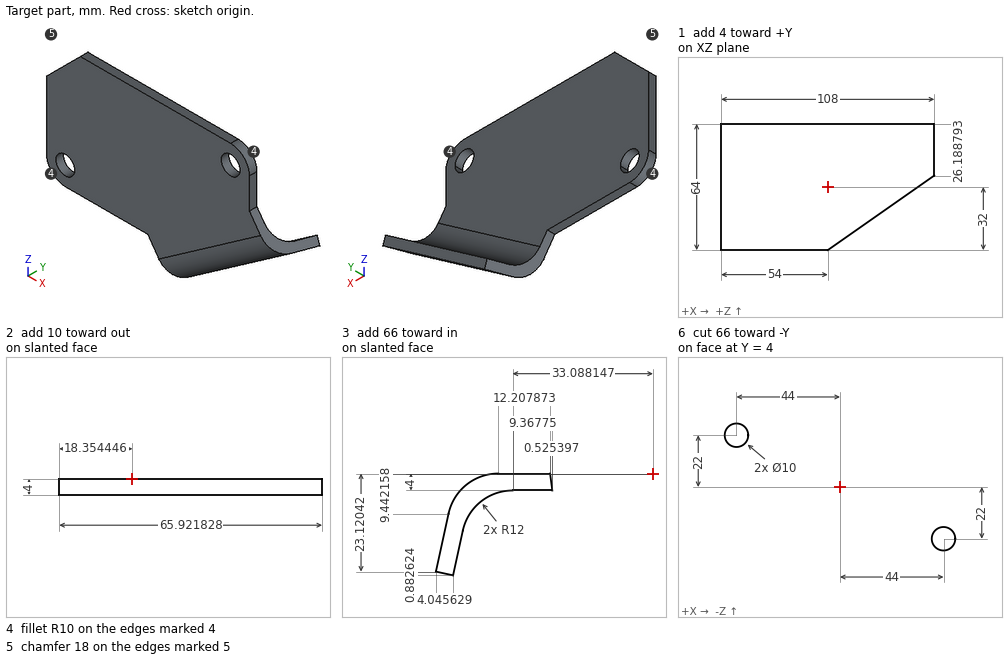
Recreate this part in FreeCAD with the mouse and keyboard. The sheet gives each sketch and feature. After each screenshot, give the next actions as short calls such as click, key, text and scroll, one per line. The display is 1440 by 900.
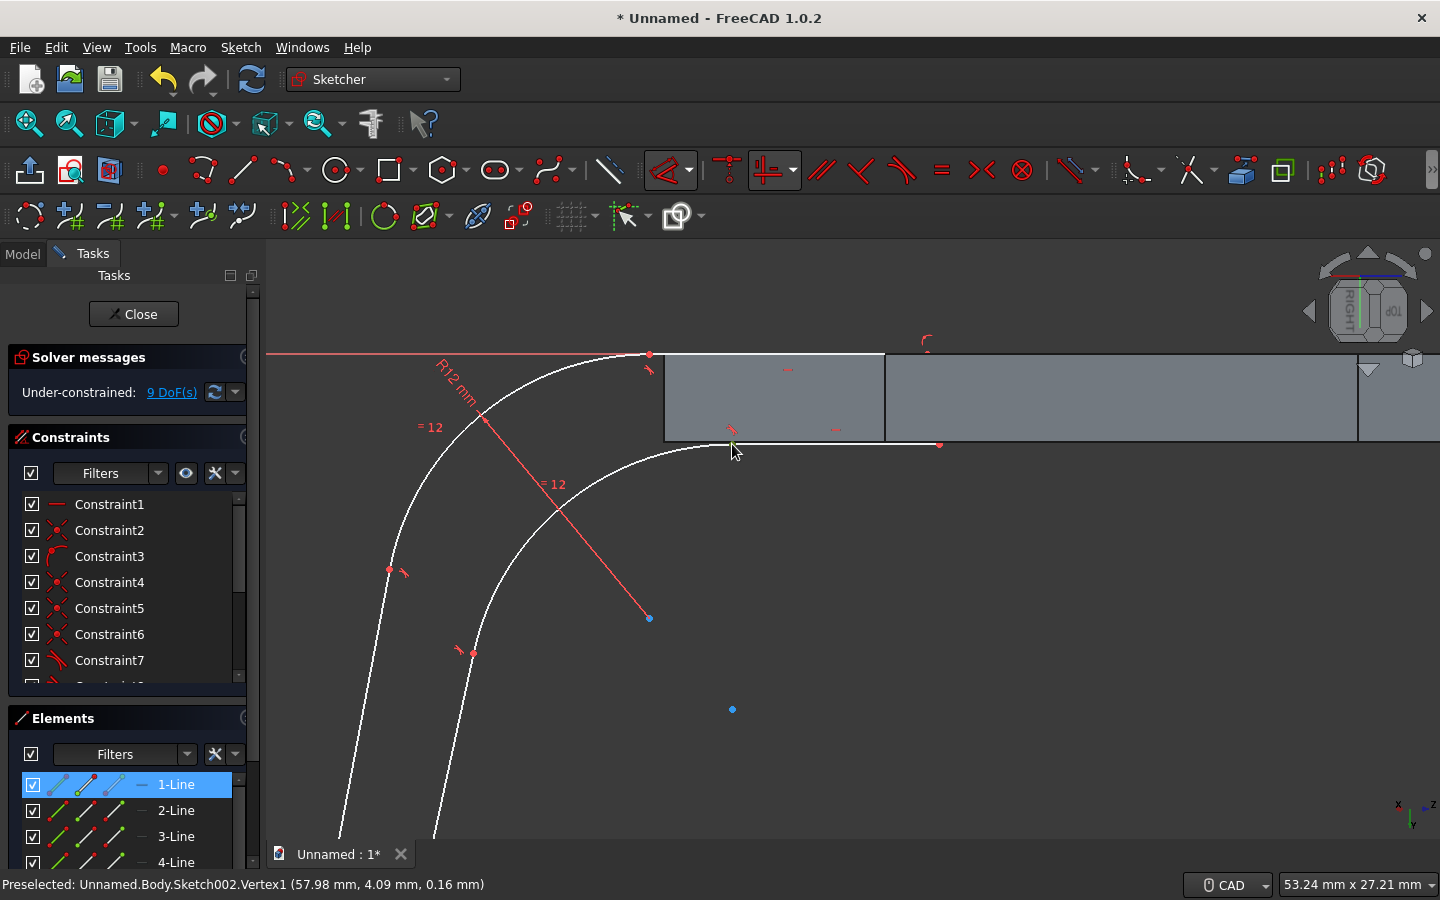
key(i)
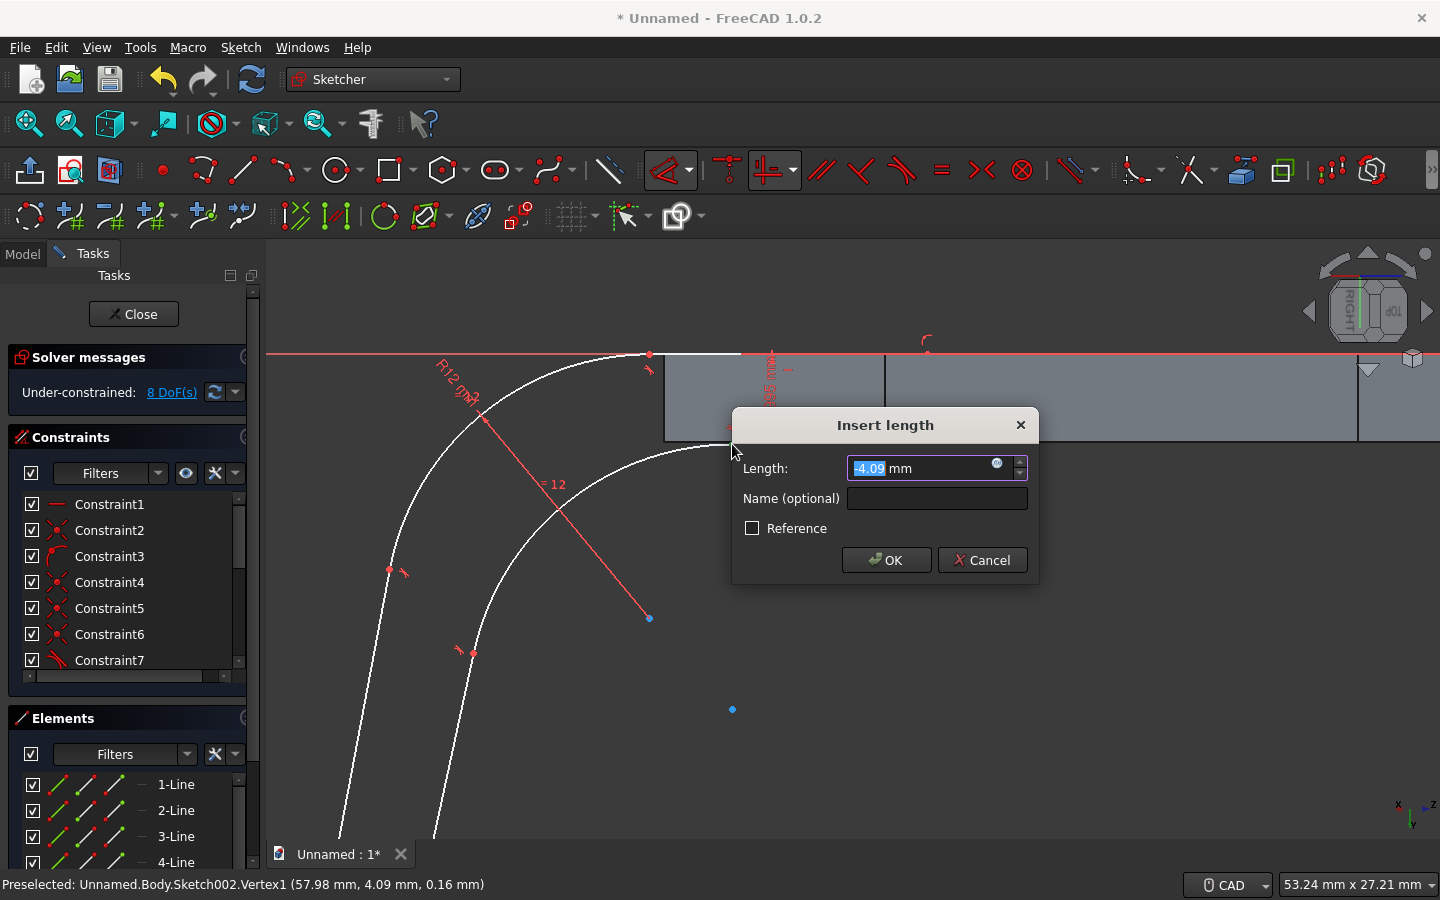
text(-4)
key(Return)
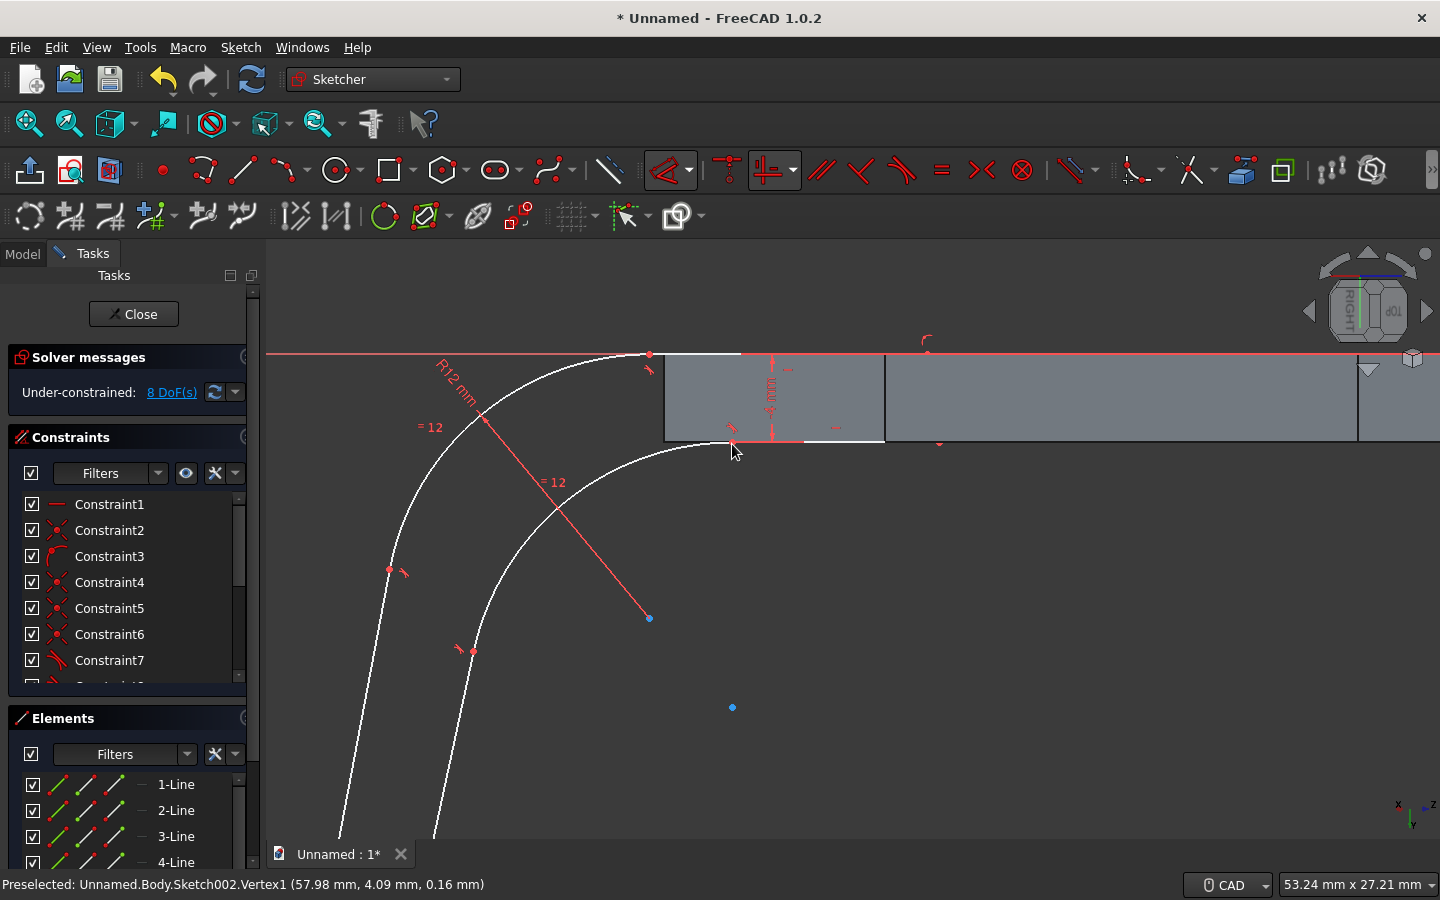
click(795, 442)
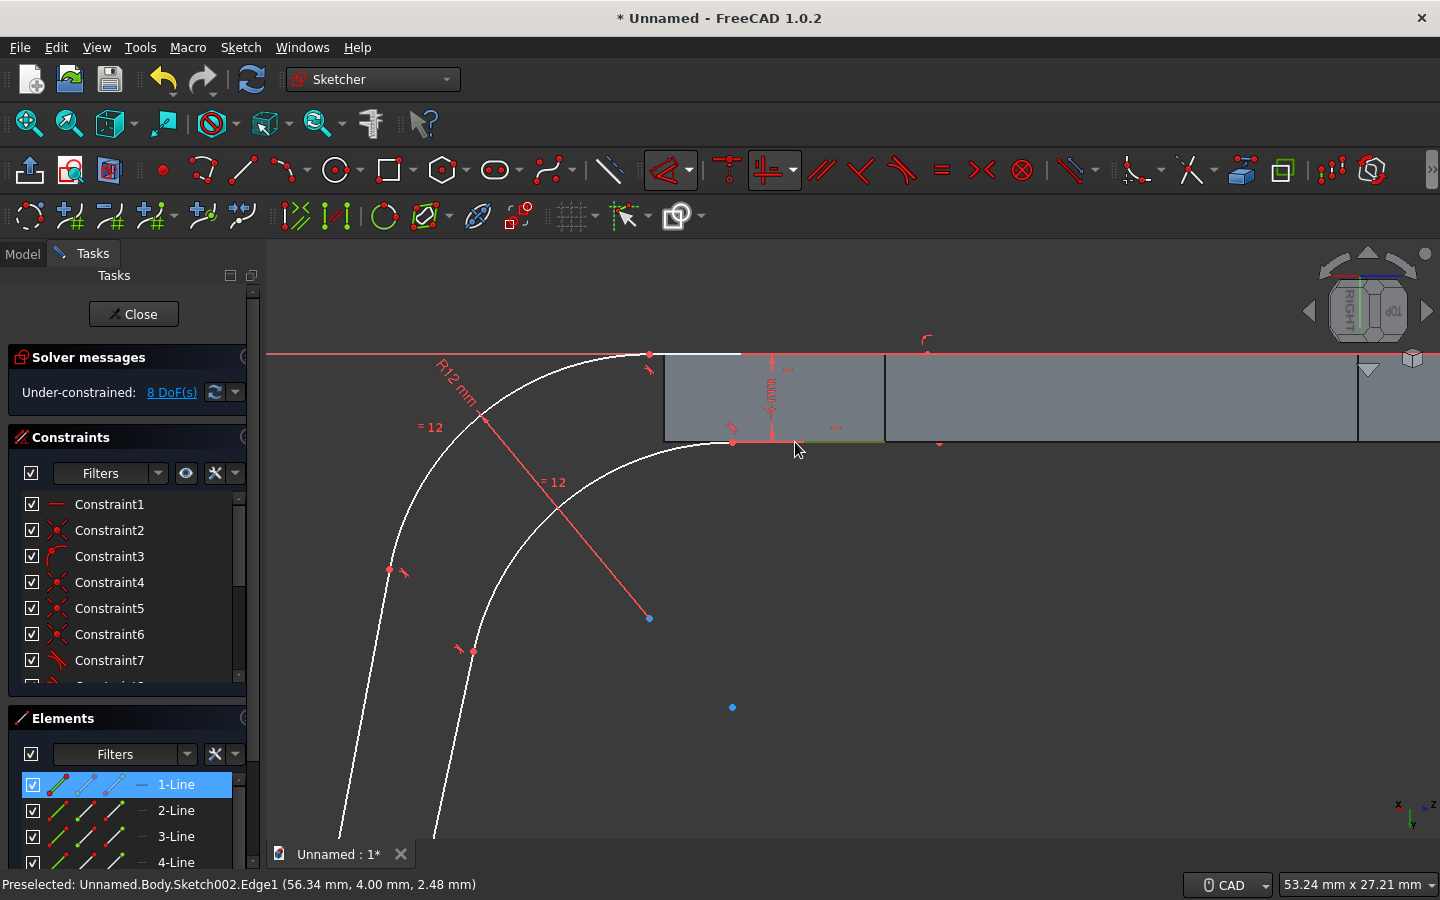
key(l)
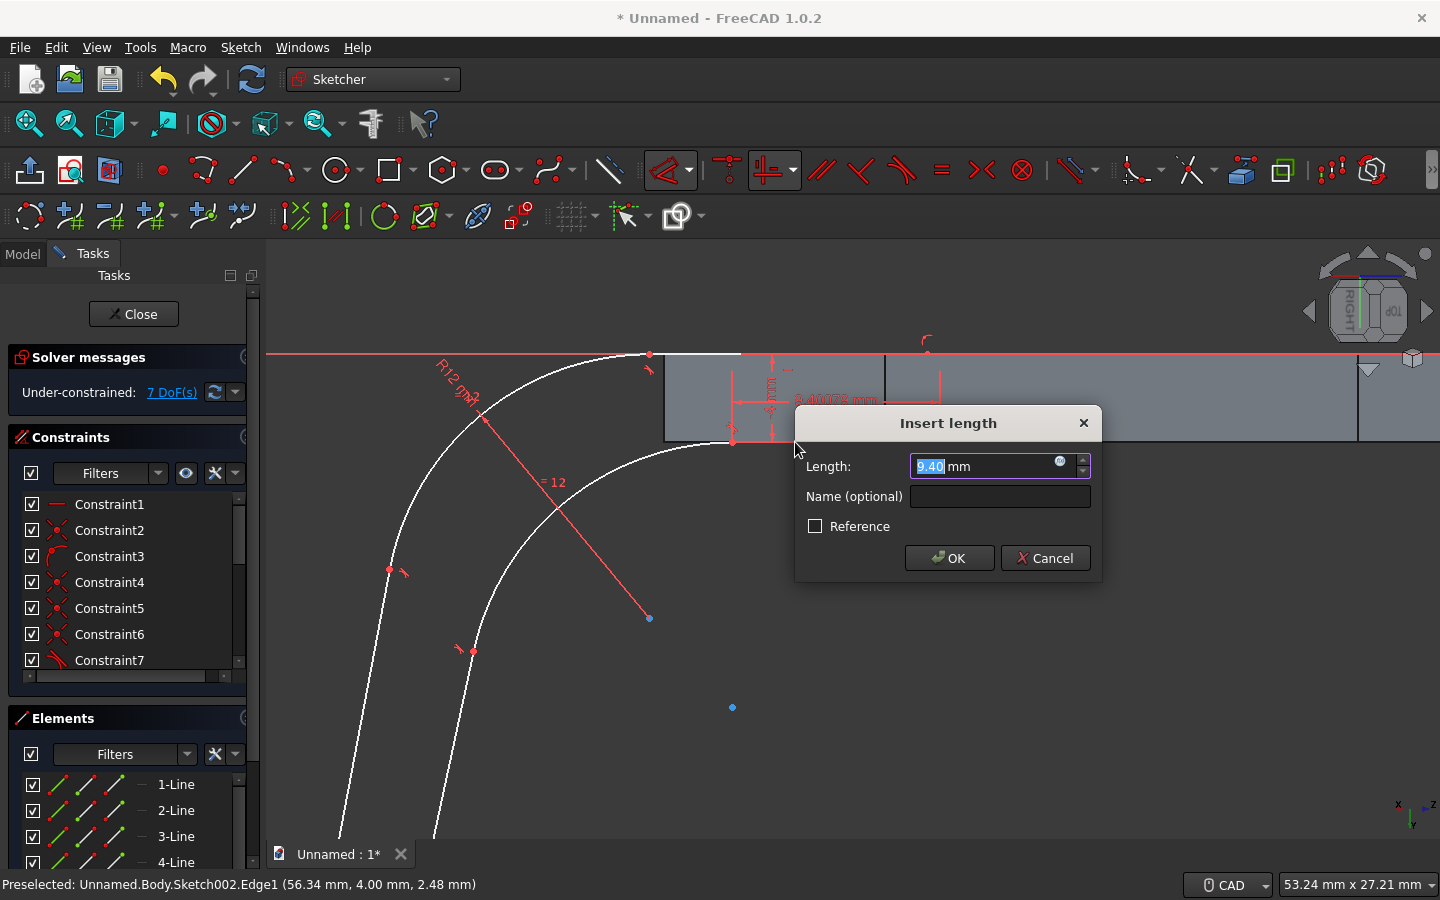
text(9.36775)
key(Return)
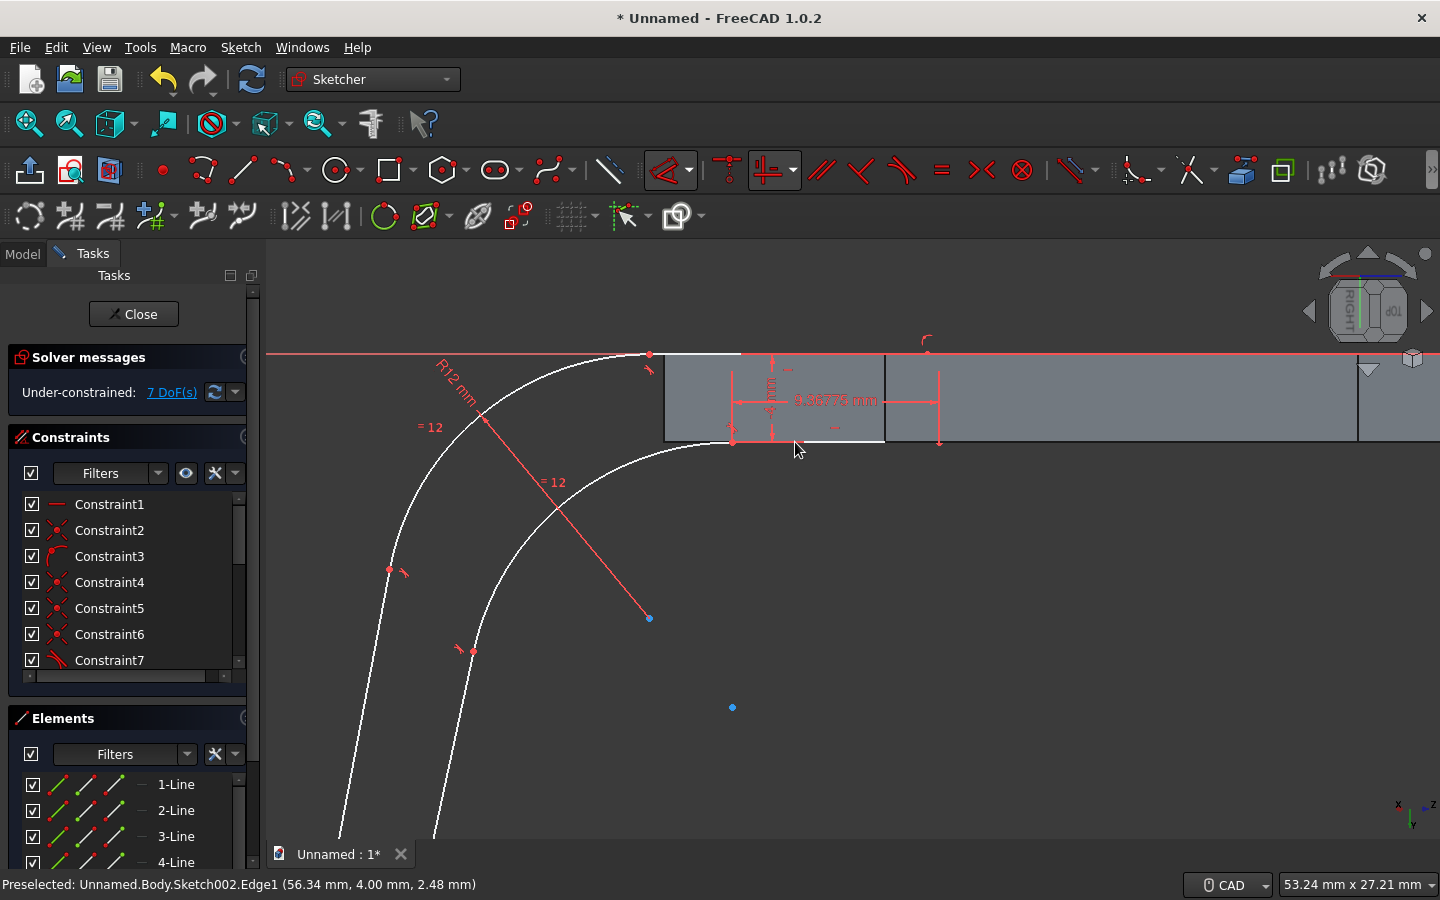
click(844, 354)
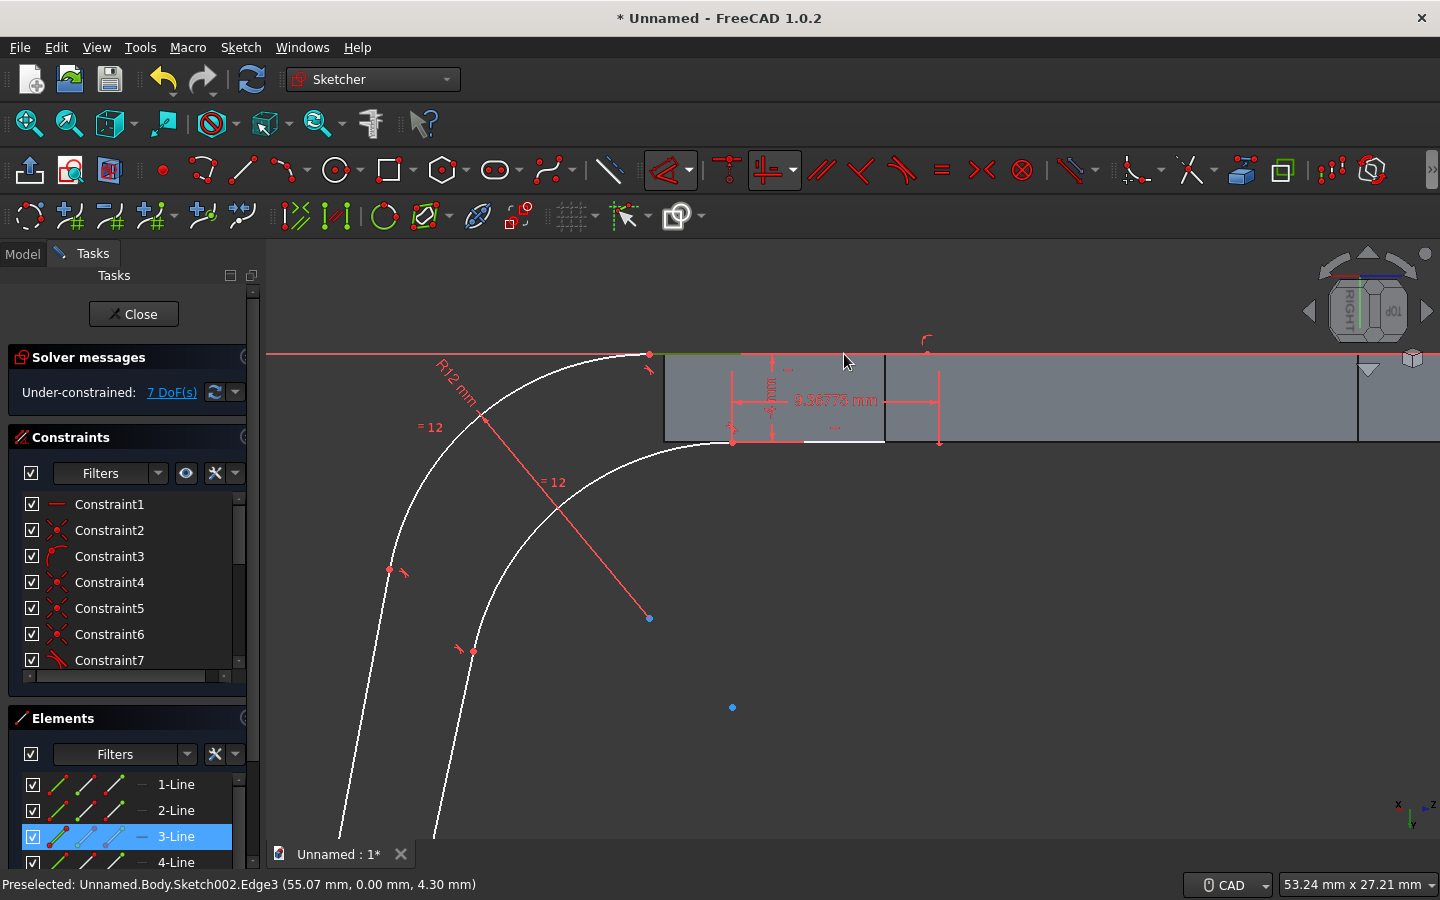
key(l)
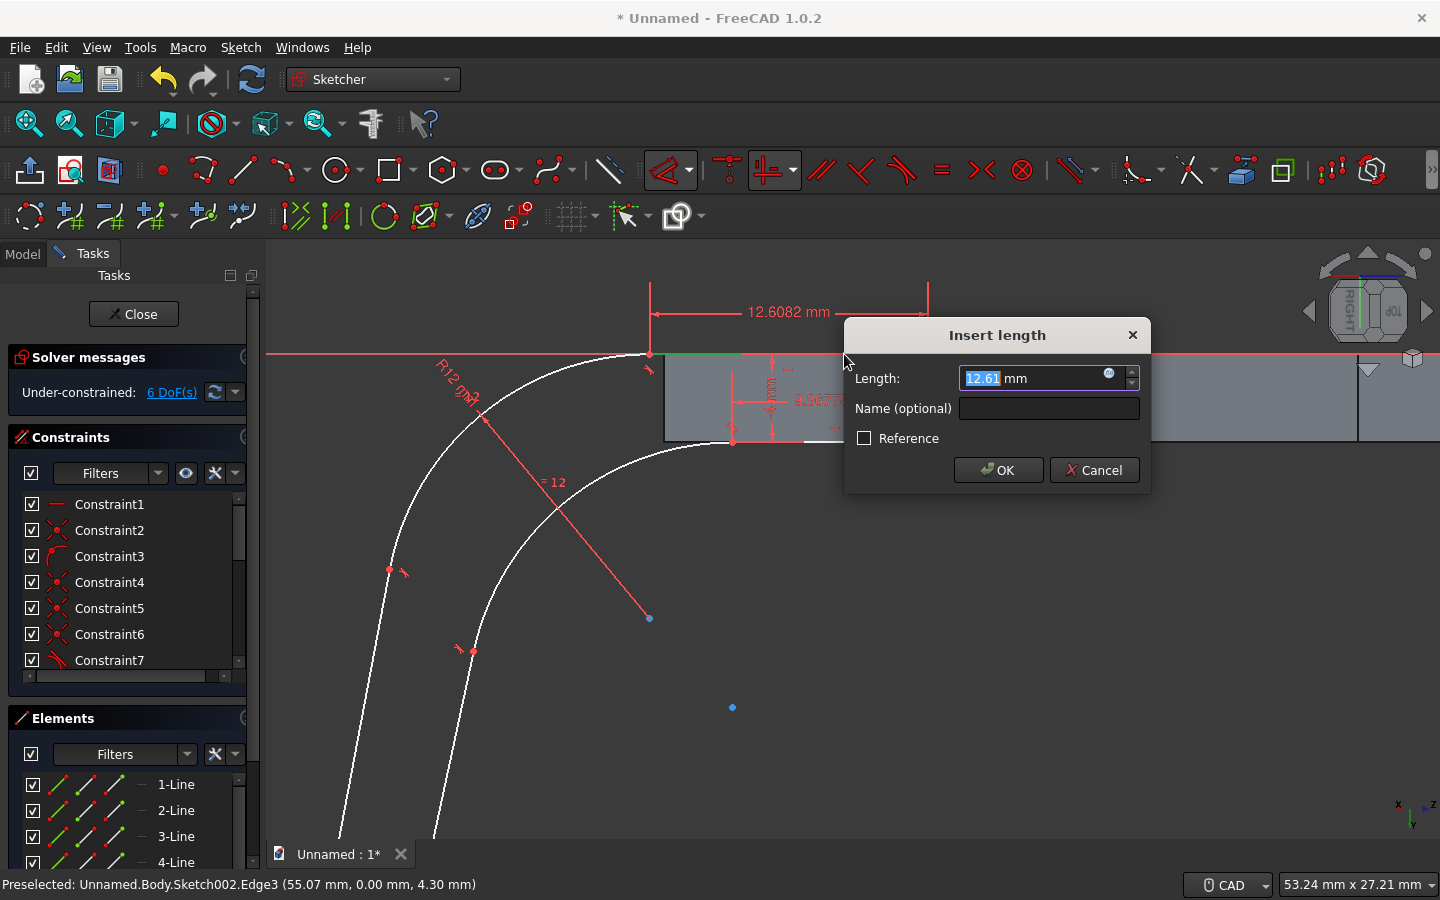
text(12.207873)
key(Return)